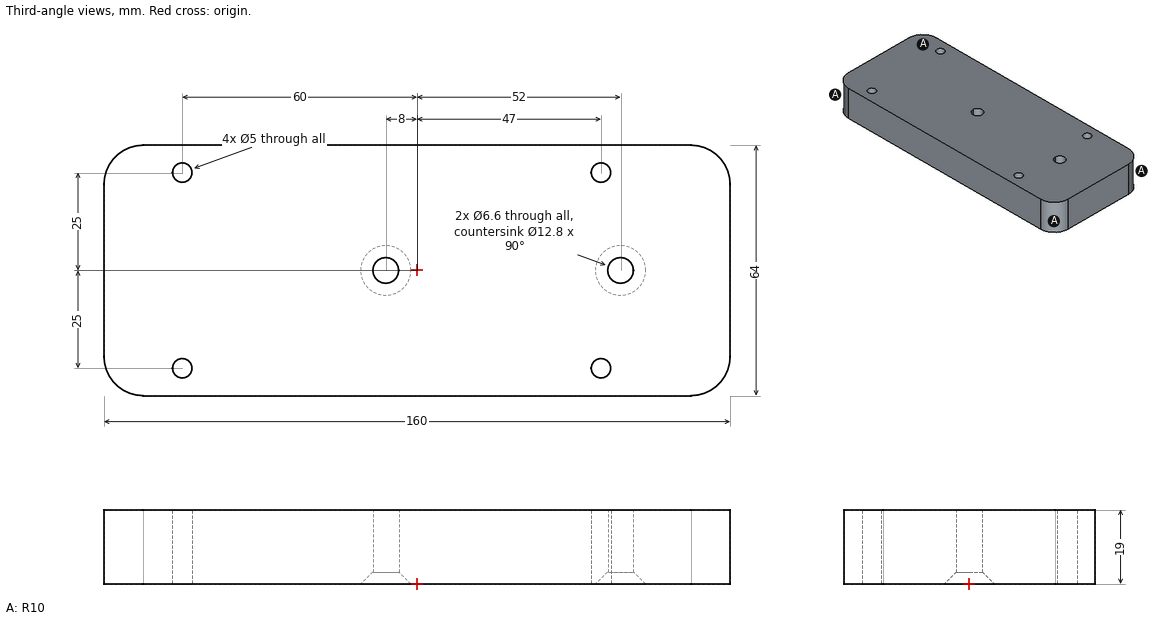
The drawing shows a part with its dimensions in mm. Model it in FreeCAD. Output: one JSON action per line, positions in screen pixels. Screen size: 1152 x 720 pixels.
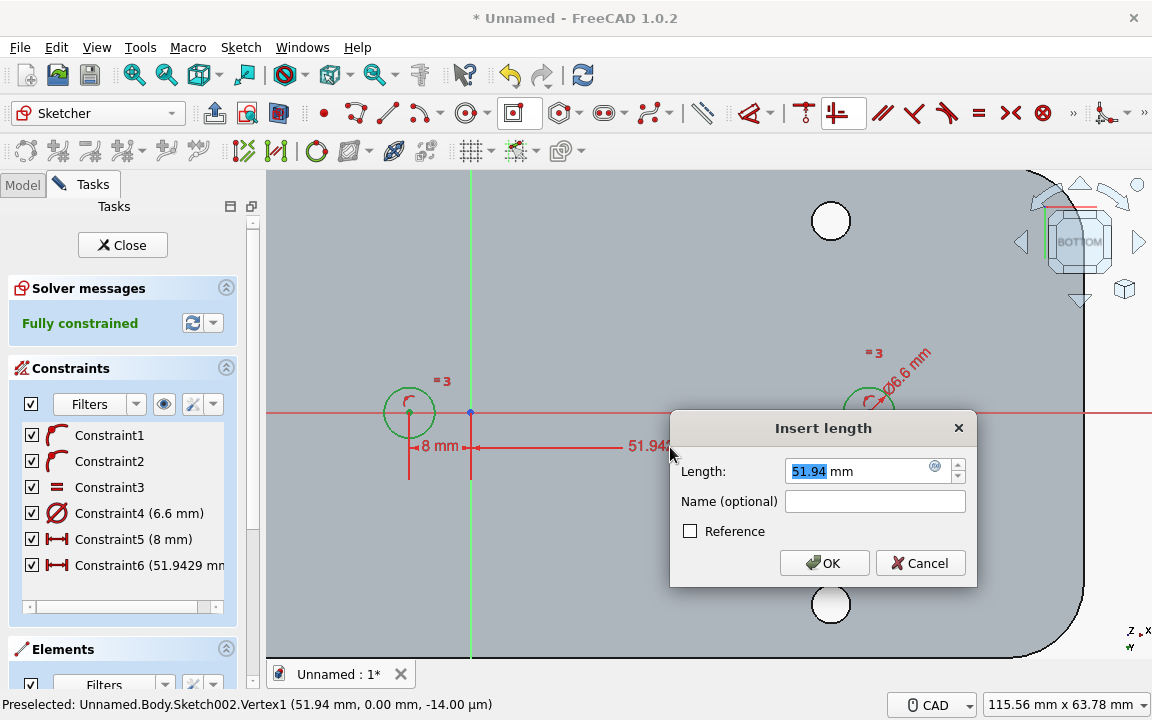
{"action": "type", "text": "52"}
{"action": "key", "text": "Return"}
{"action": "key", "text": "Escape"}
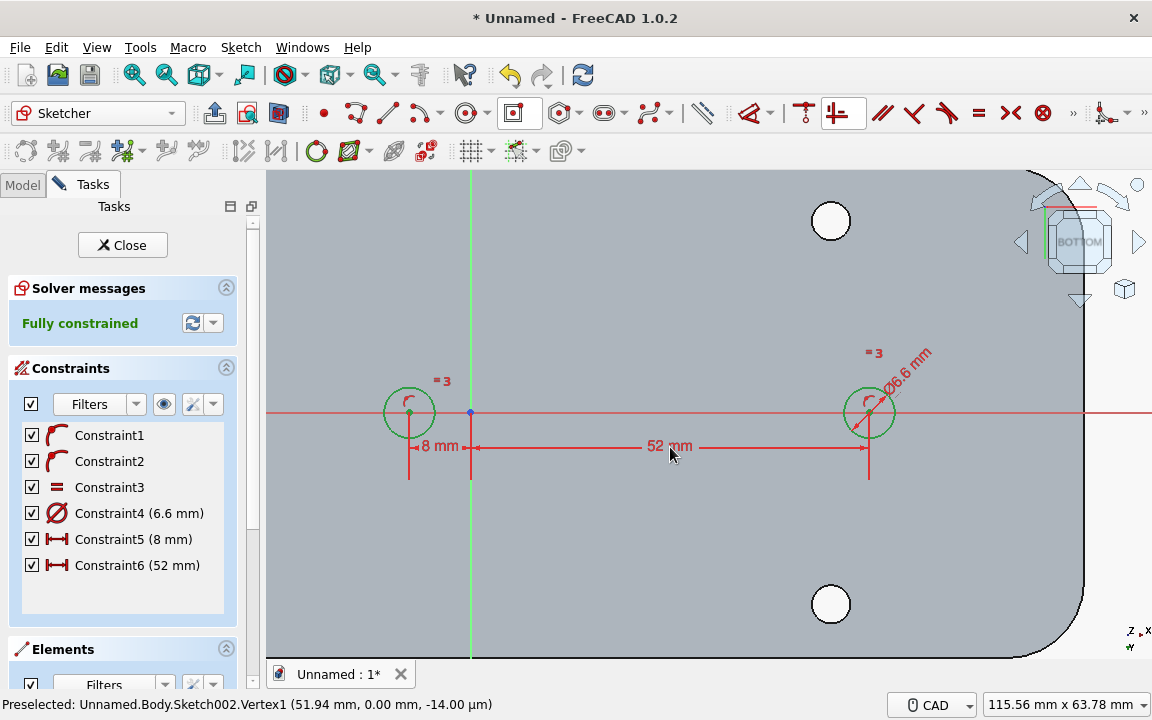
{"action": "left_click", "coordinate": [123, 245]}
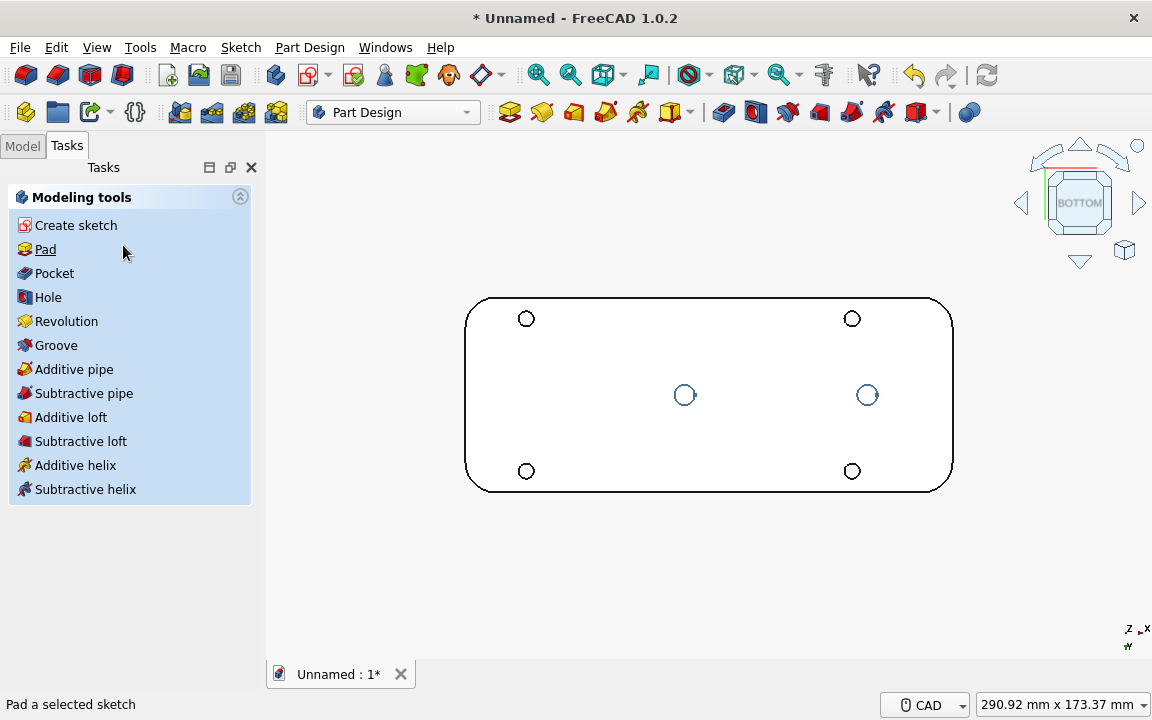
{"action": "left_click", "coordinate": [756, 112]}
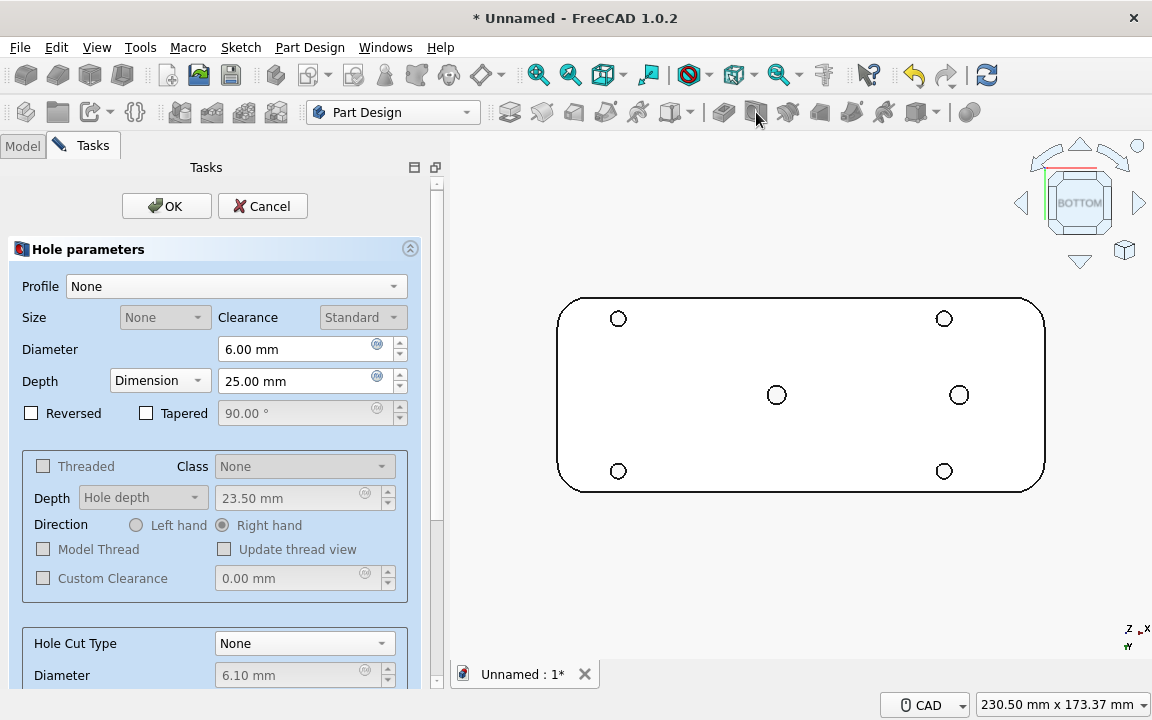
{"action": "triple_click", "coordinate": [305, 349]}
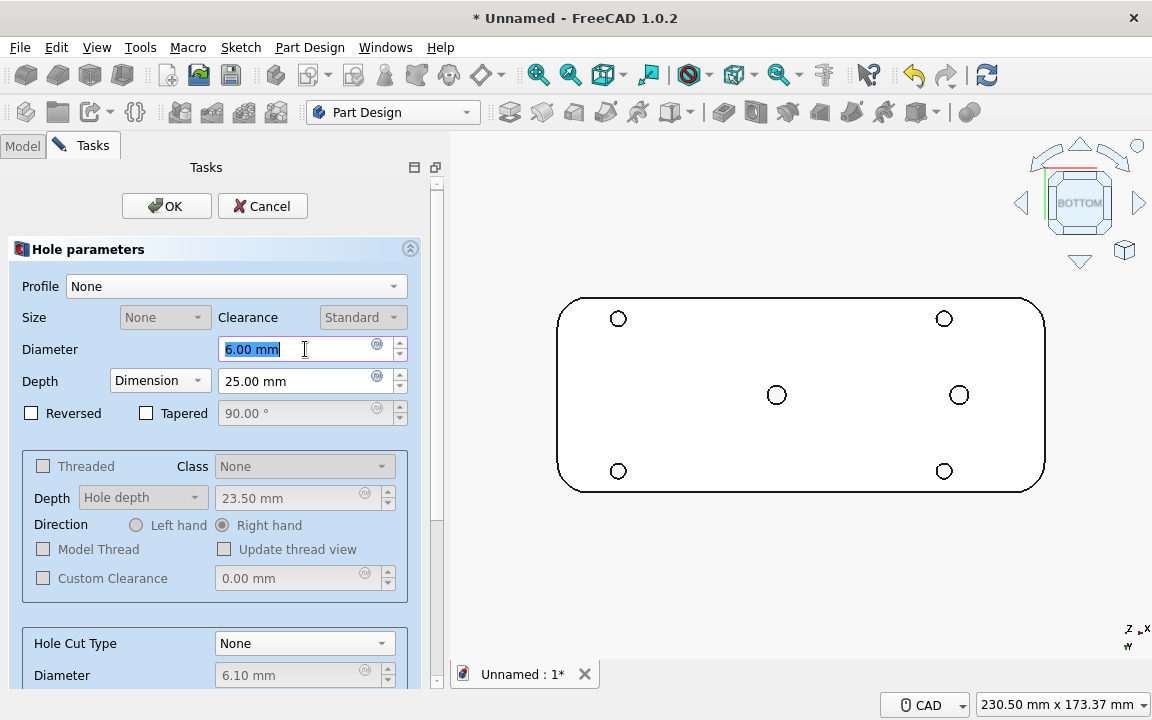
{"action": "type", "text": "6.6"}
{"action": "key", "text": "Tab"}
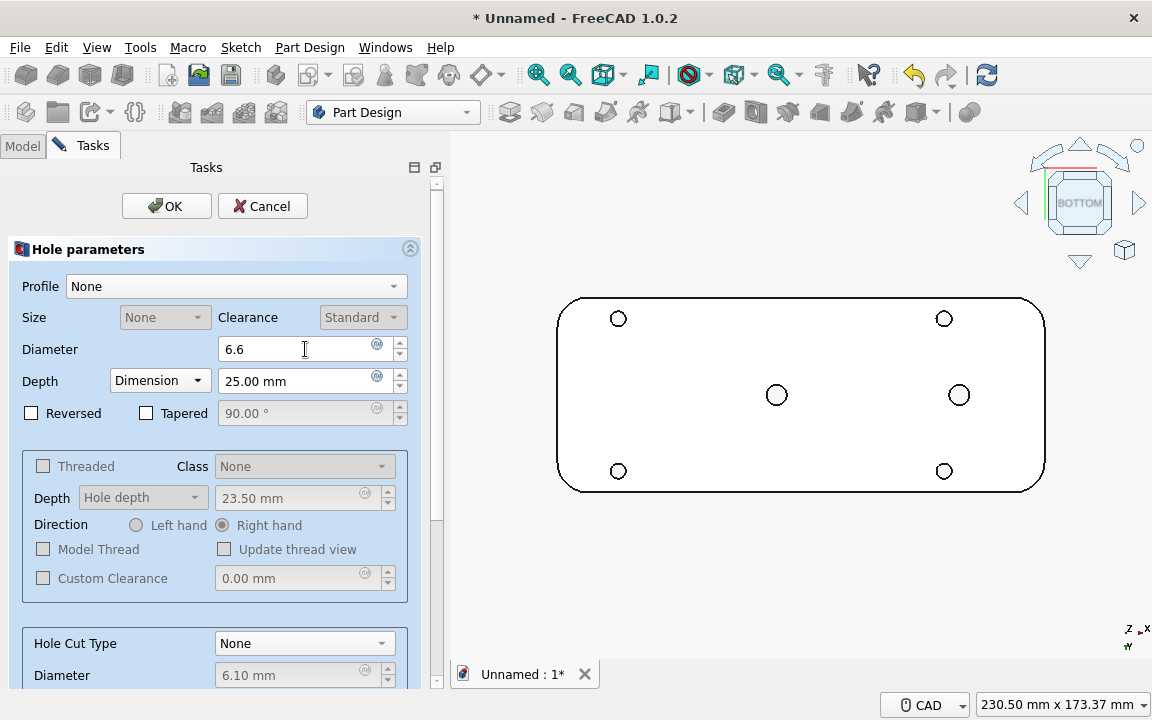
{"action": "left_click", "coordinate": [161, 380]}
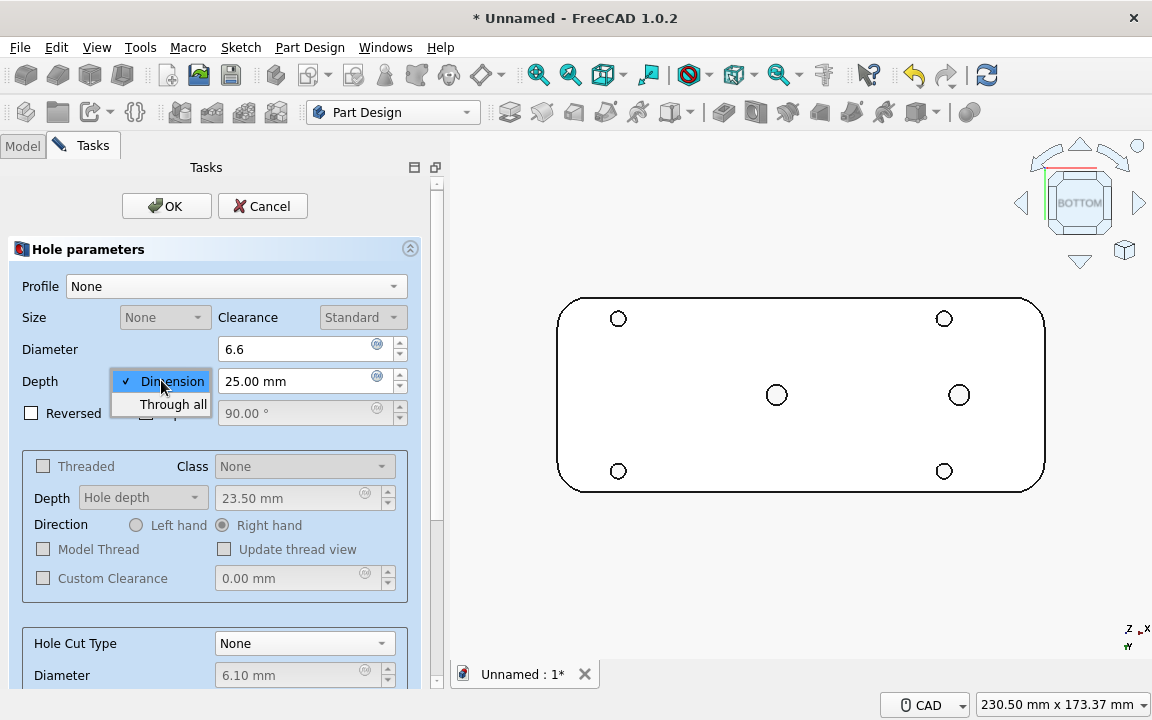
{"action": "left_click", "coordinate": [160, 404]}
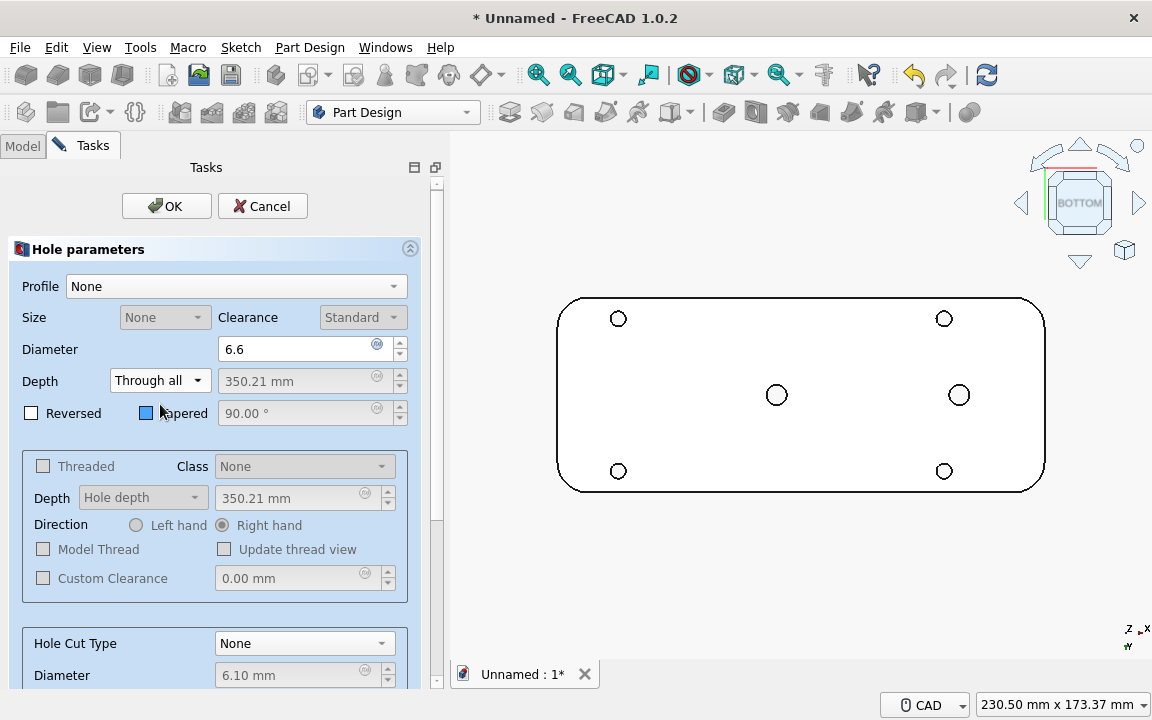
{"action": "left_click", "coordinate": [306, 644]}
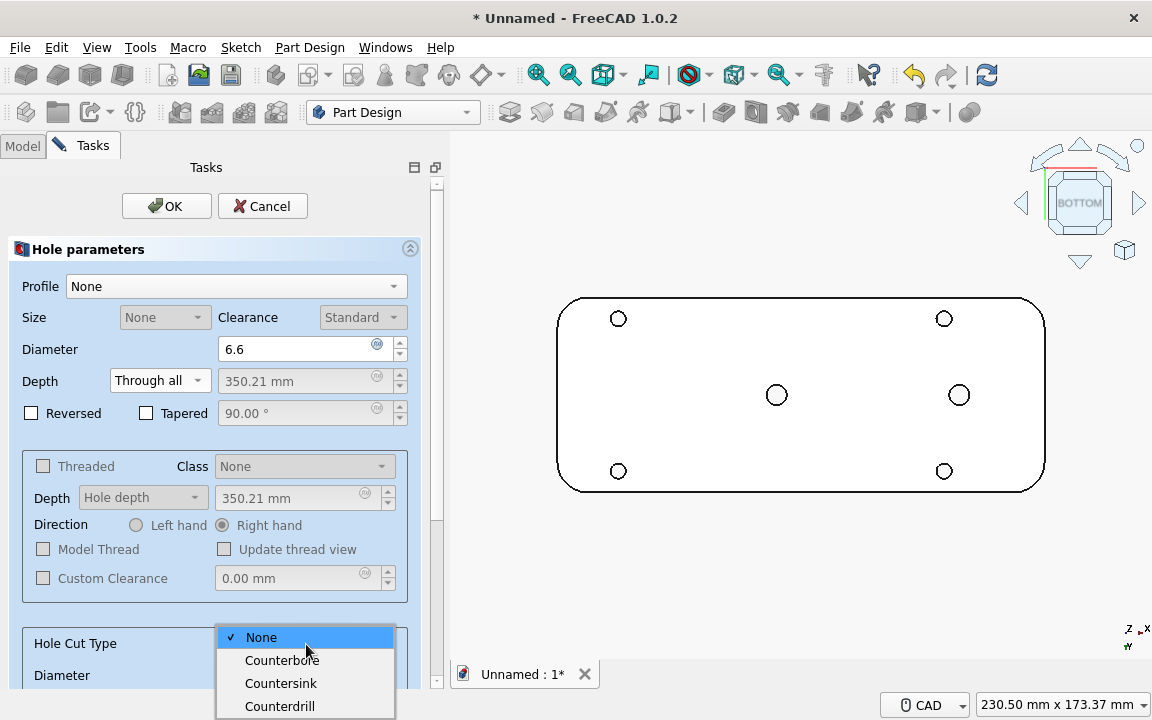
{"action": "left_click", "coordinate": [304, 684]}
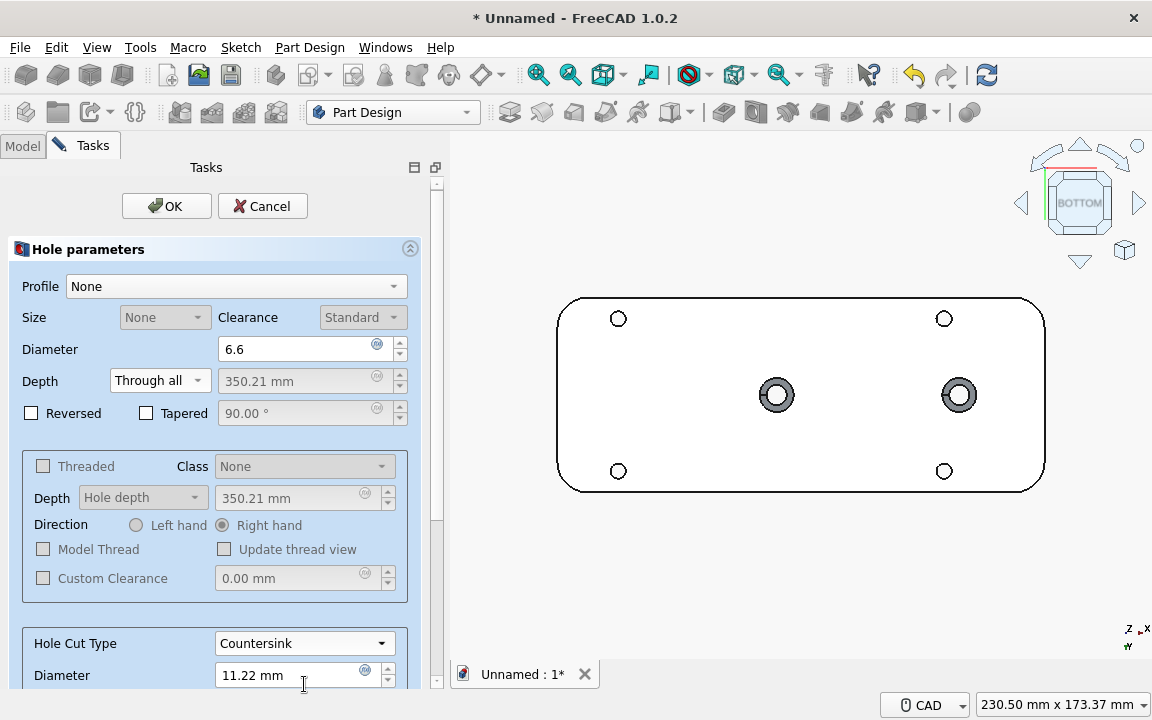
{"action": "triple_click", "coordinate": [298, 675]}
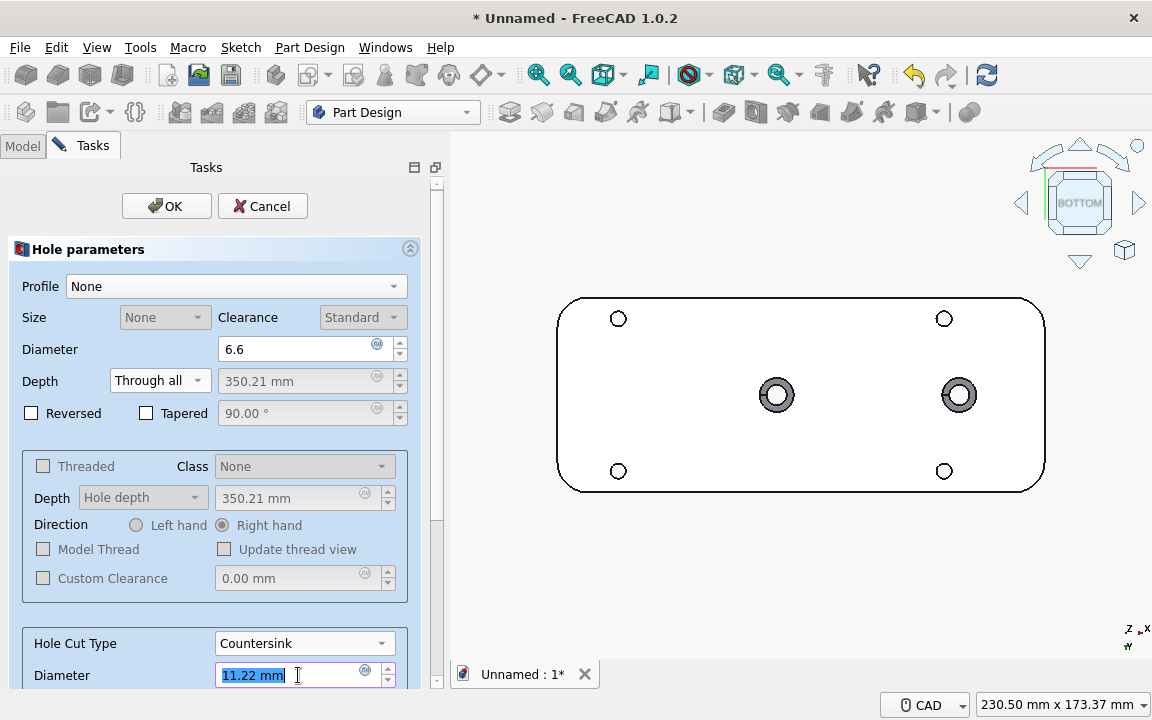
{"action": "type", "text": "12.8"}
{"action": "key", "text": "Tab"}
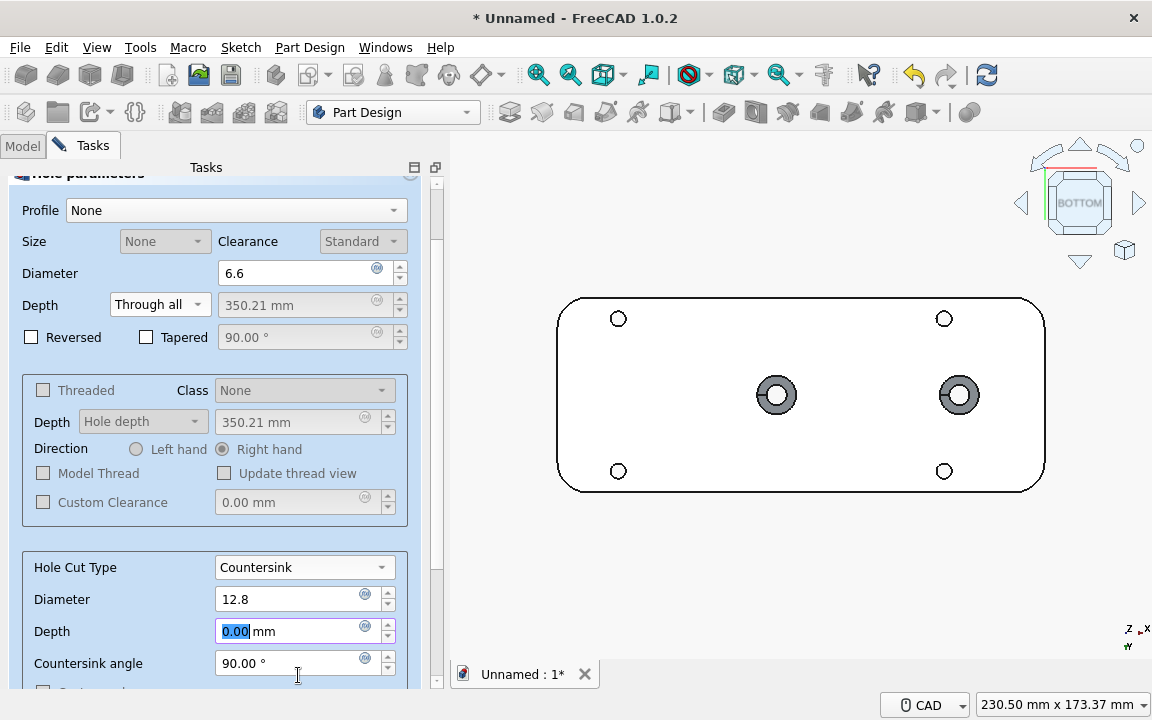
{"action": "scroll", "coordinate": [437, 432], "scroll_direction": "up", "scroll_amount": 3}